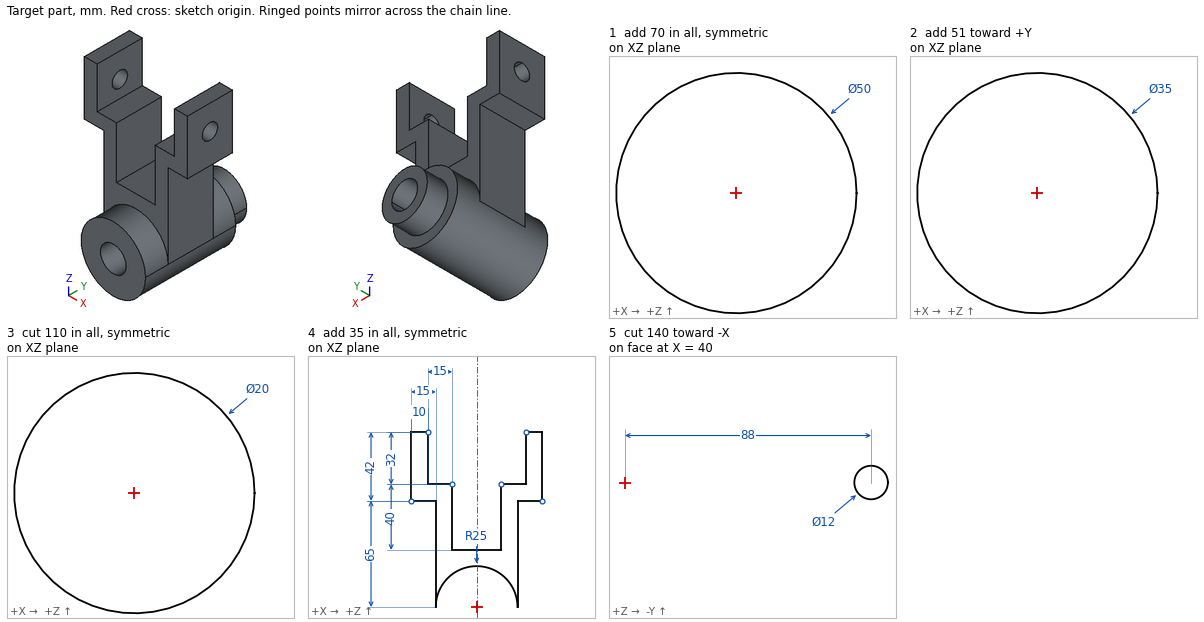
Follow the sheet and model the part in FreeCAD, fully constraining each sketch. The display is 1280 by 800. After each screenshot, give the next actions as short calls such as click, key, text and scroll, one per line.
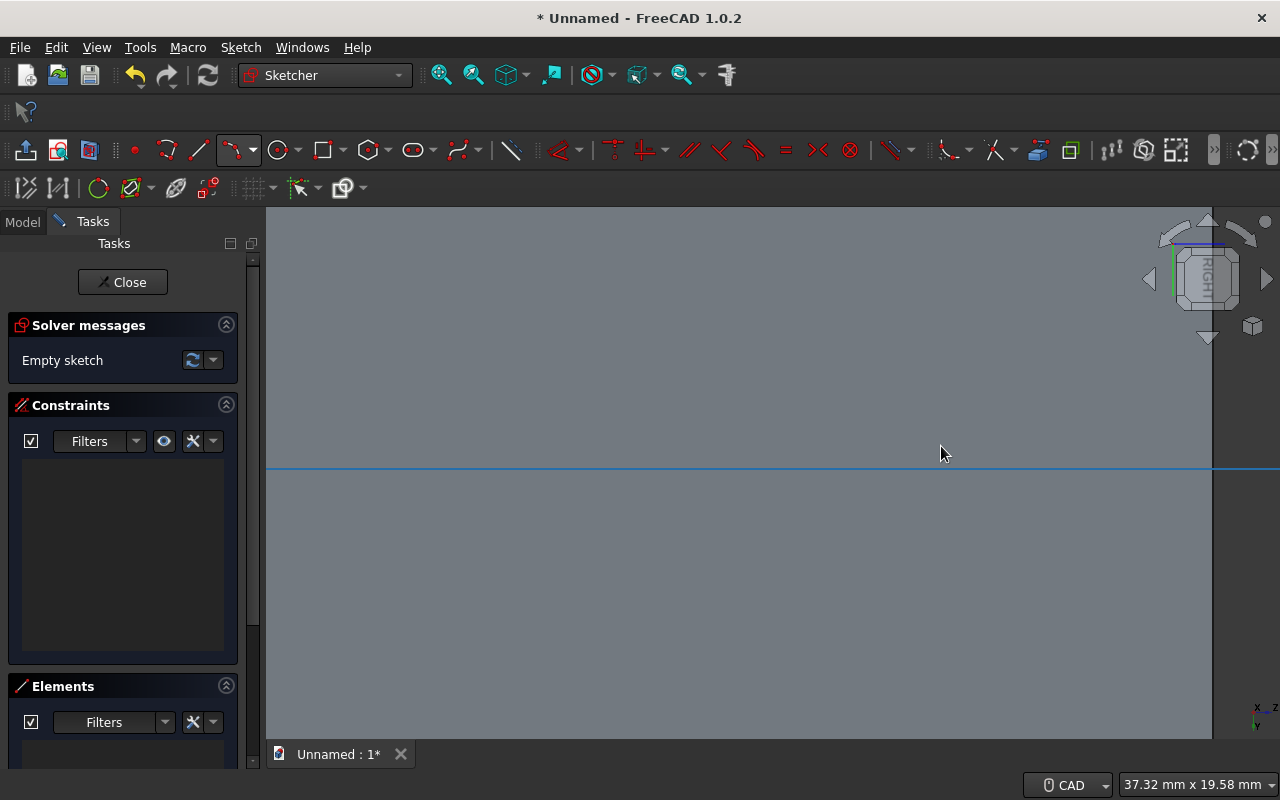
click(278, 150)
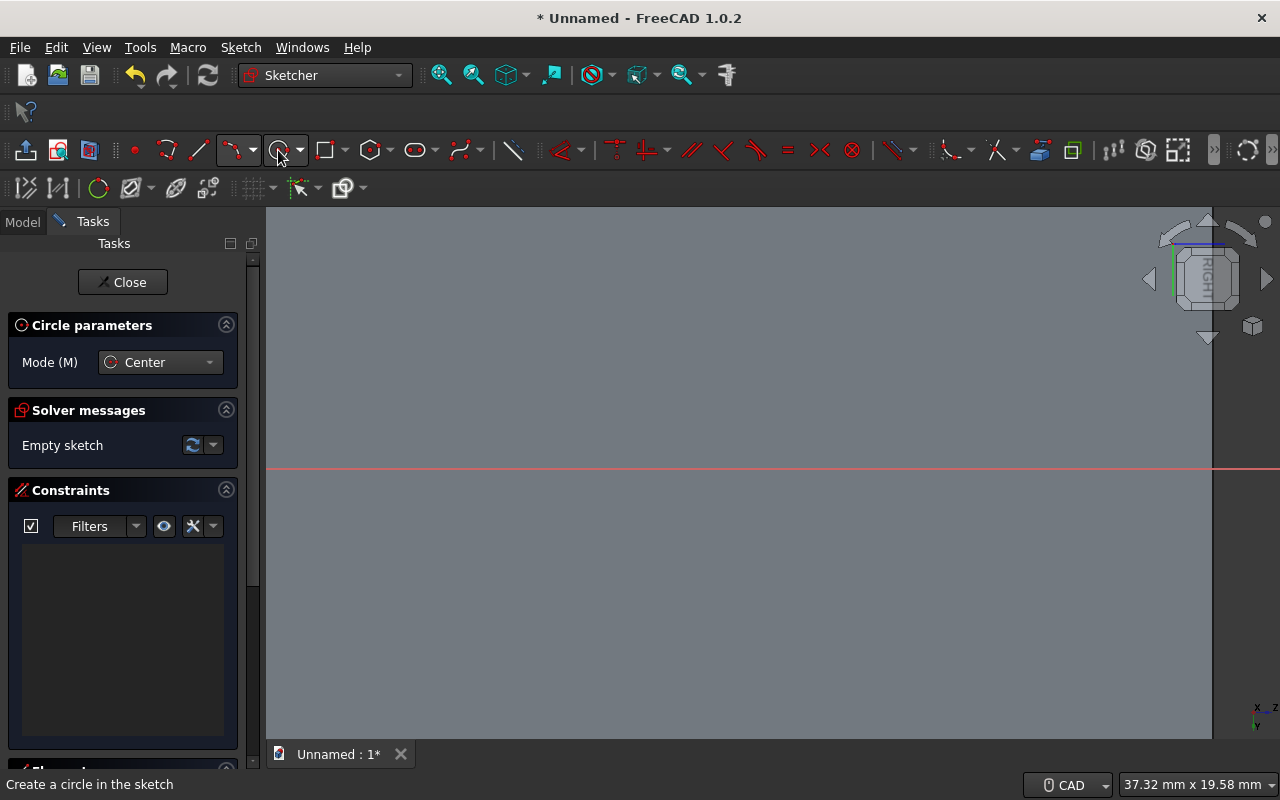
click(697, 469)
click(812, 353)
key(Escape)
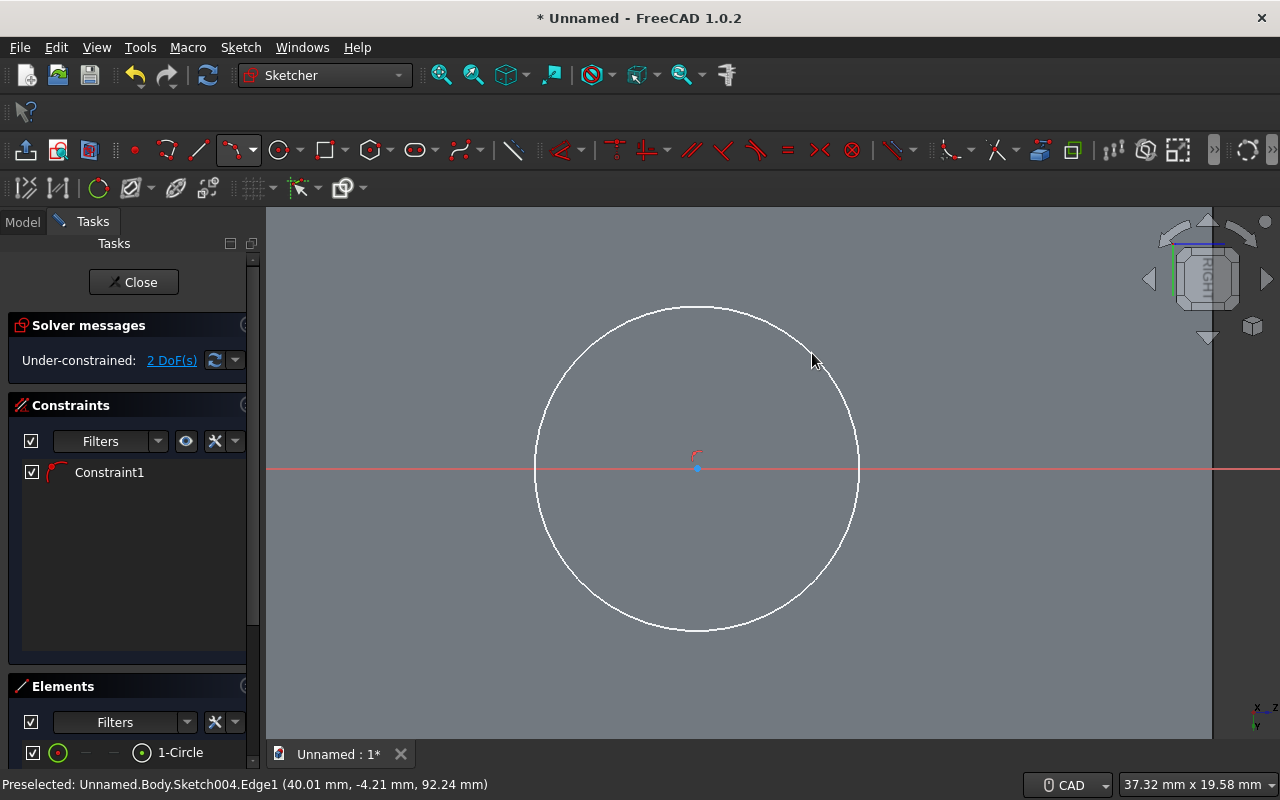
key(d)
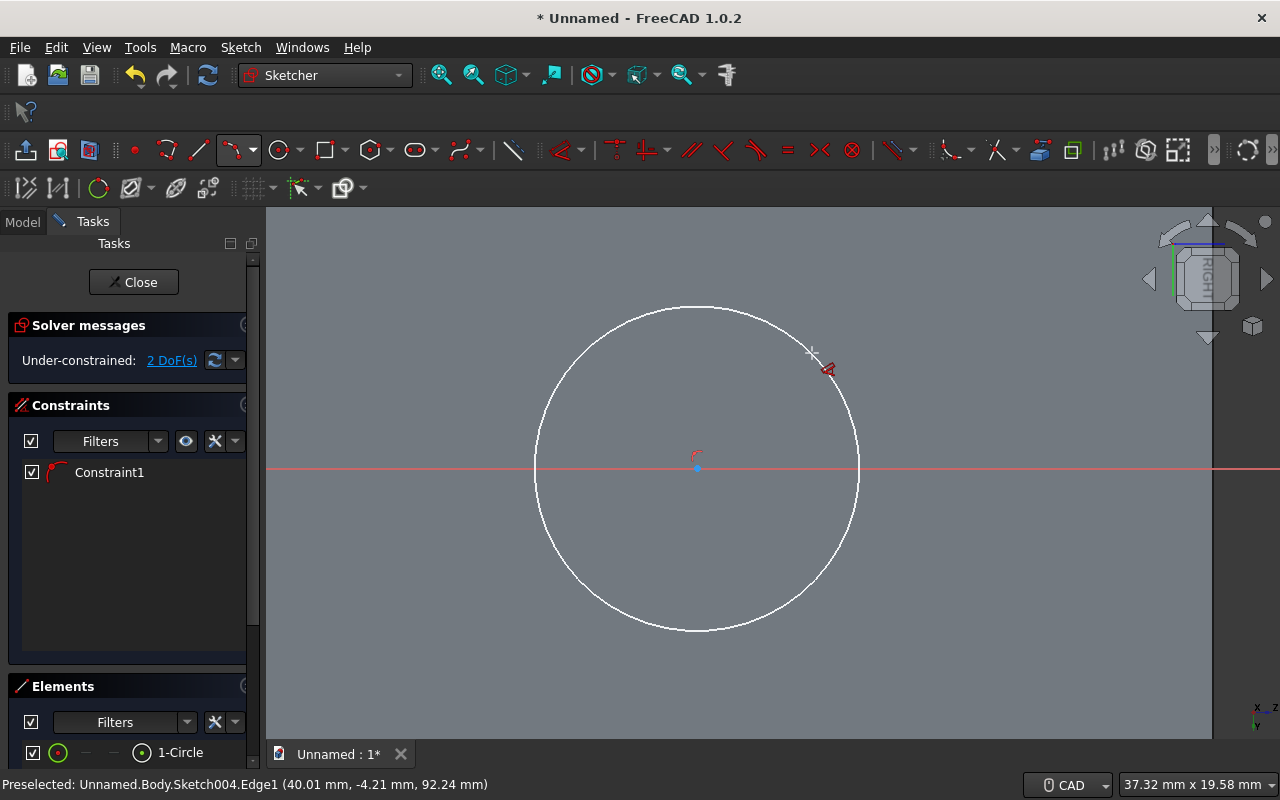
click(811, 353)
click(833, 330)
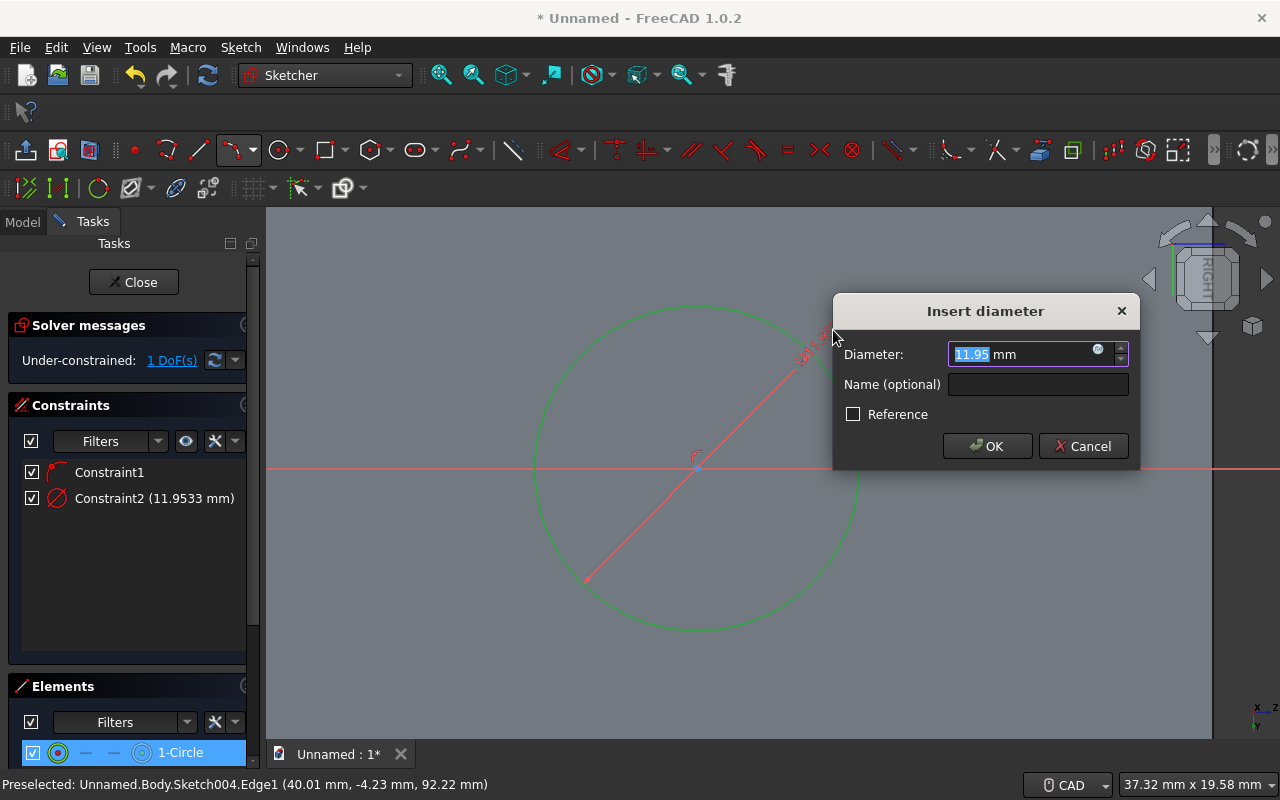
text(12)
key(Return)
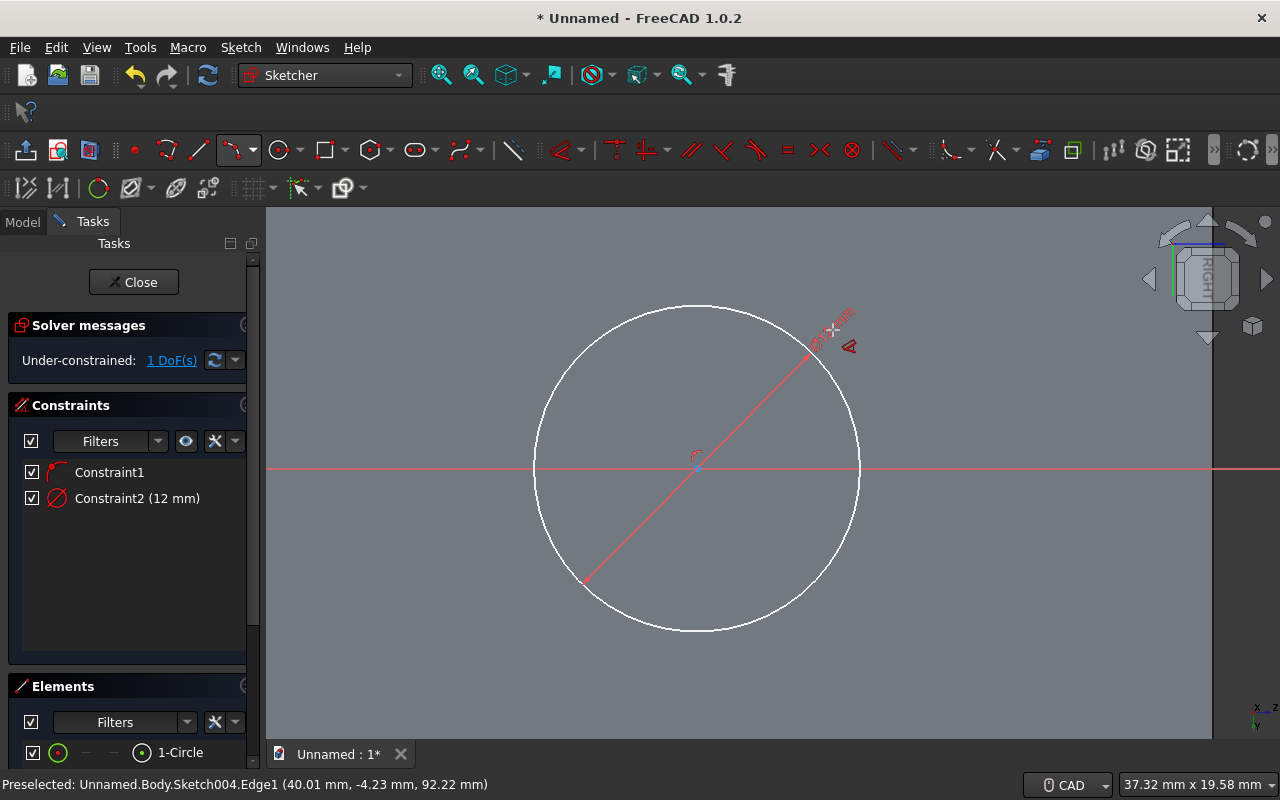
click(697, 469)
click(496, 503)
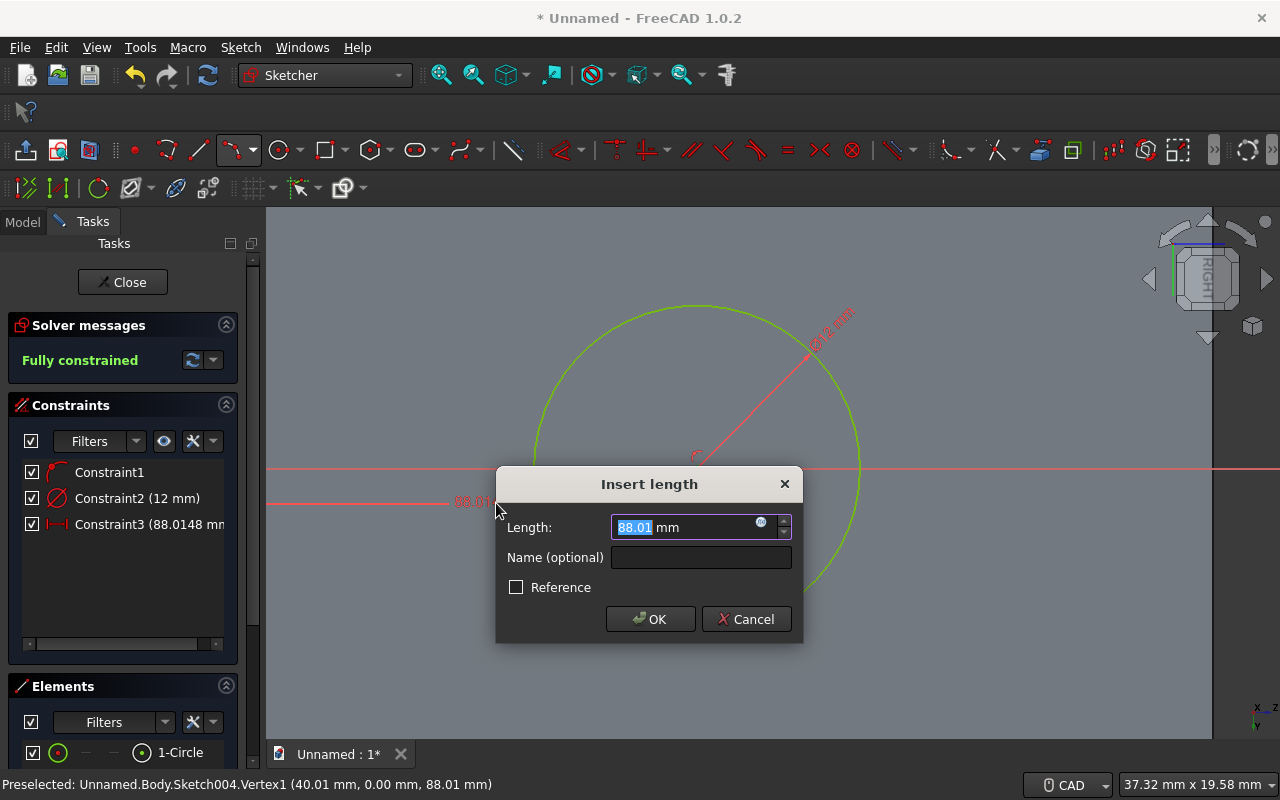
text(88)
key(Return)
key(Escape)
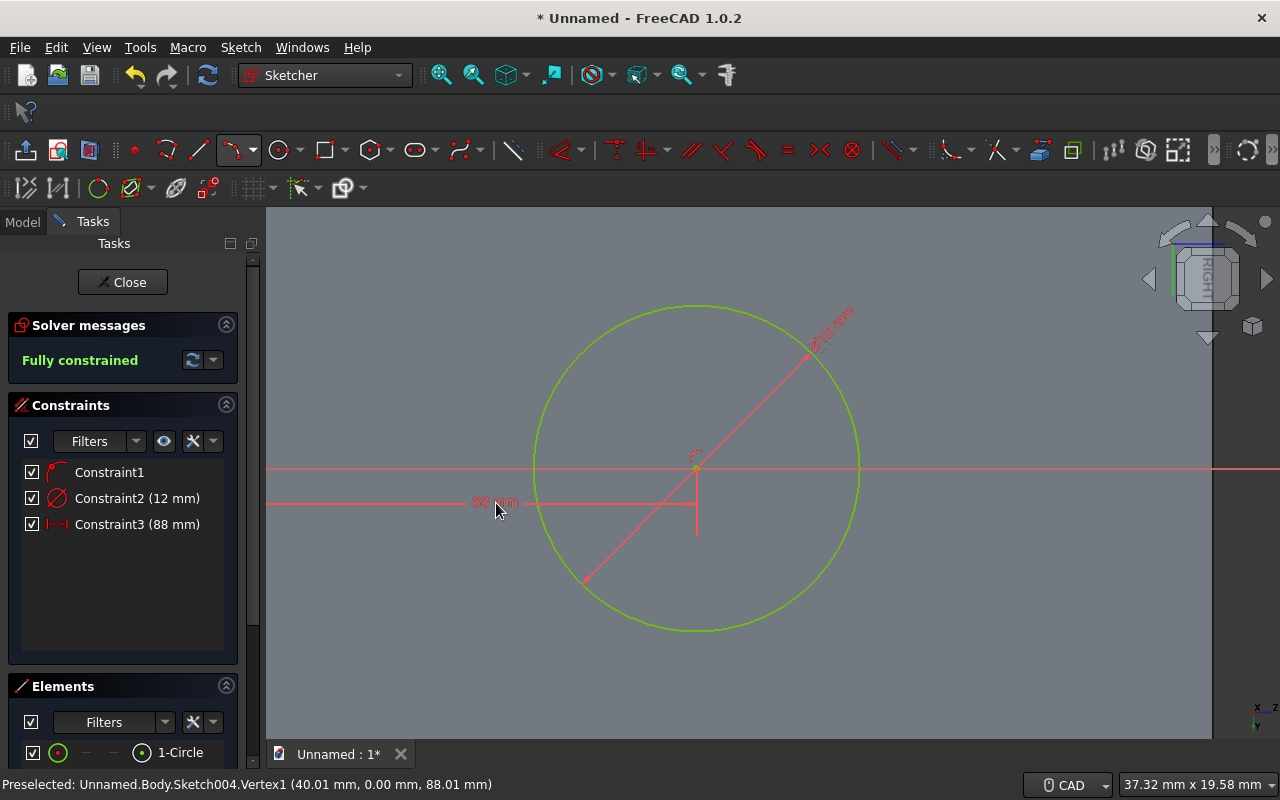
click(123, 282)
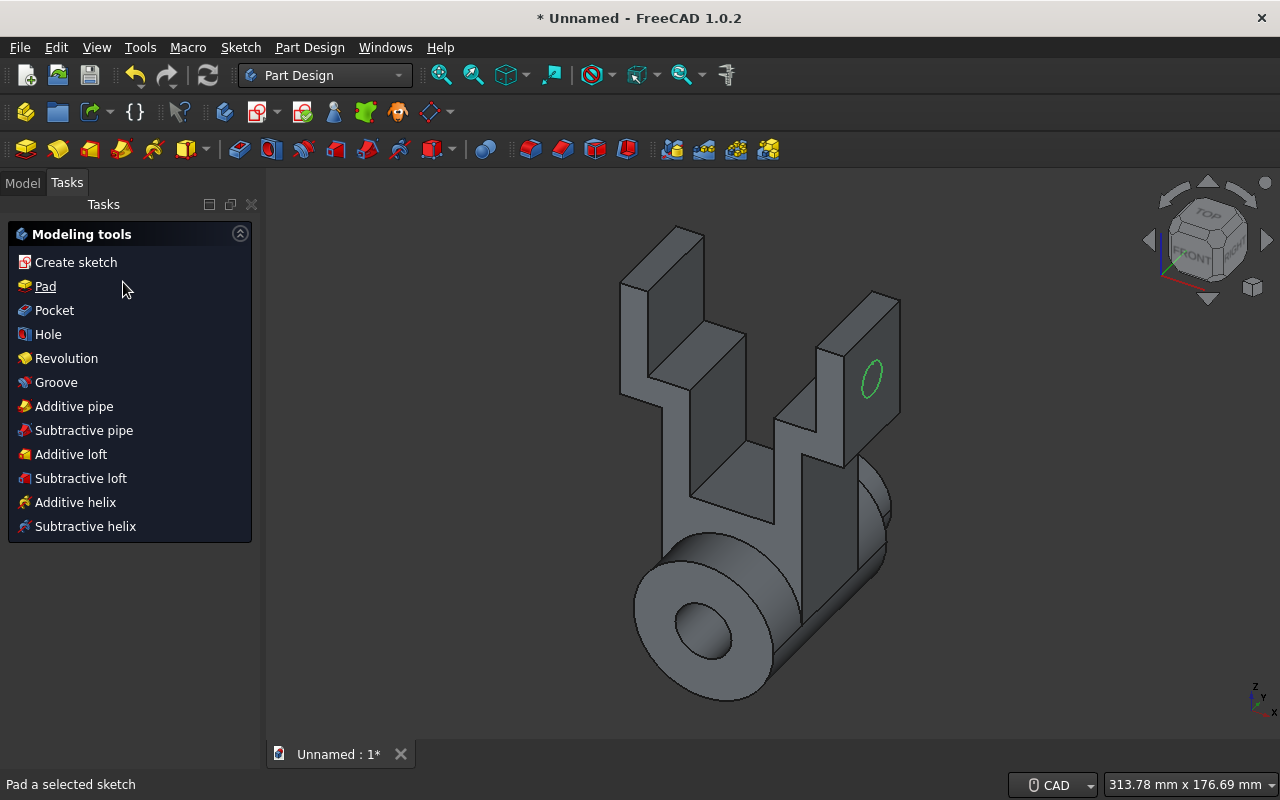
click(240, 150)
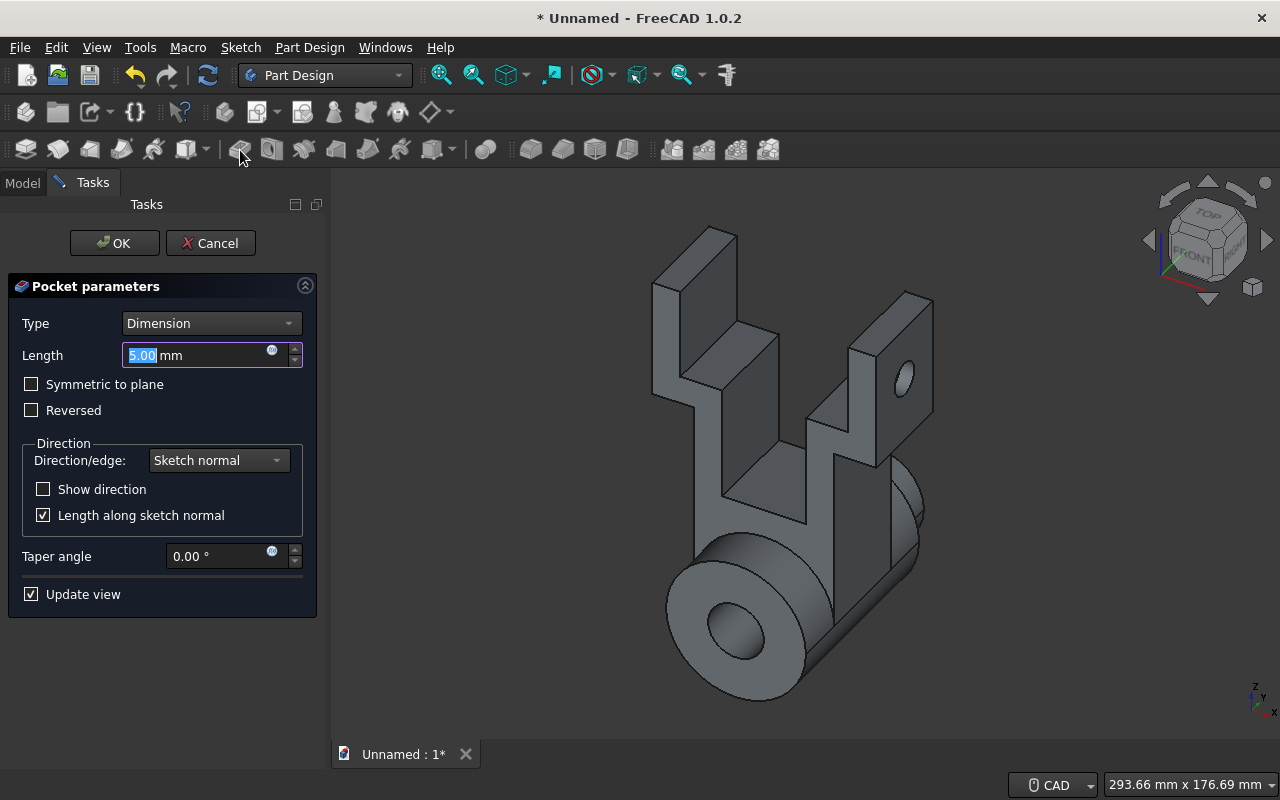
text(140)
key(Tab)